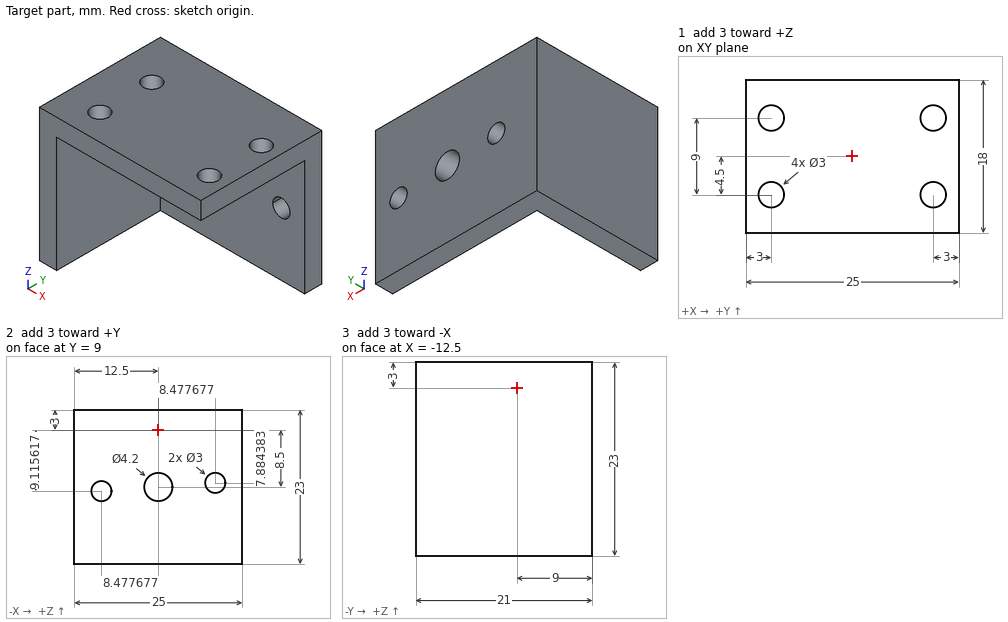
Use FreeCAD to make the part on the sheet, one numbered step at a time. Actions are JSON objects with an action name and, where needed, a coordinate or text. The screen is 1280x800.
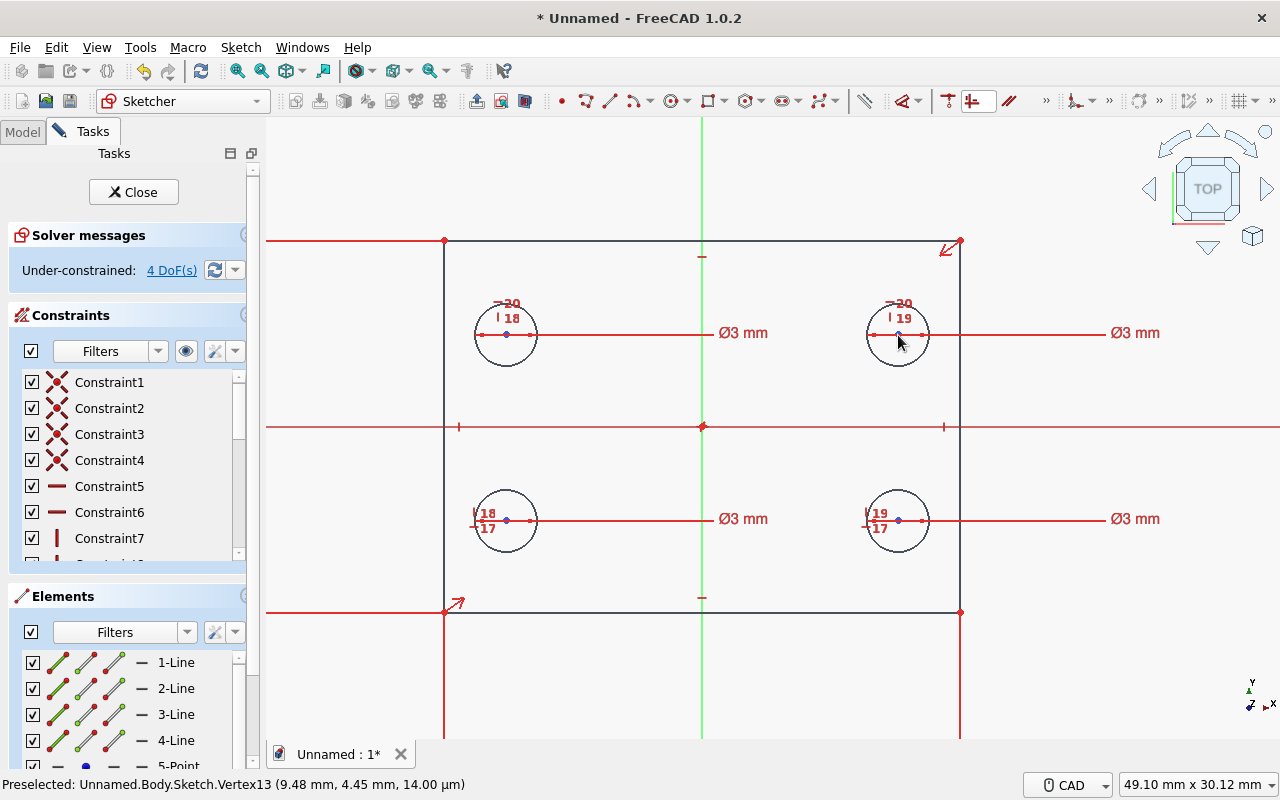
{"action": "key", "text": "d"}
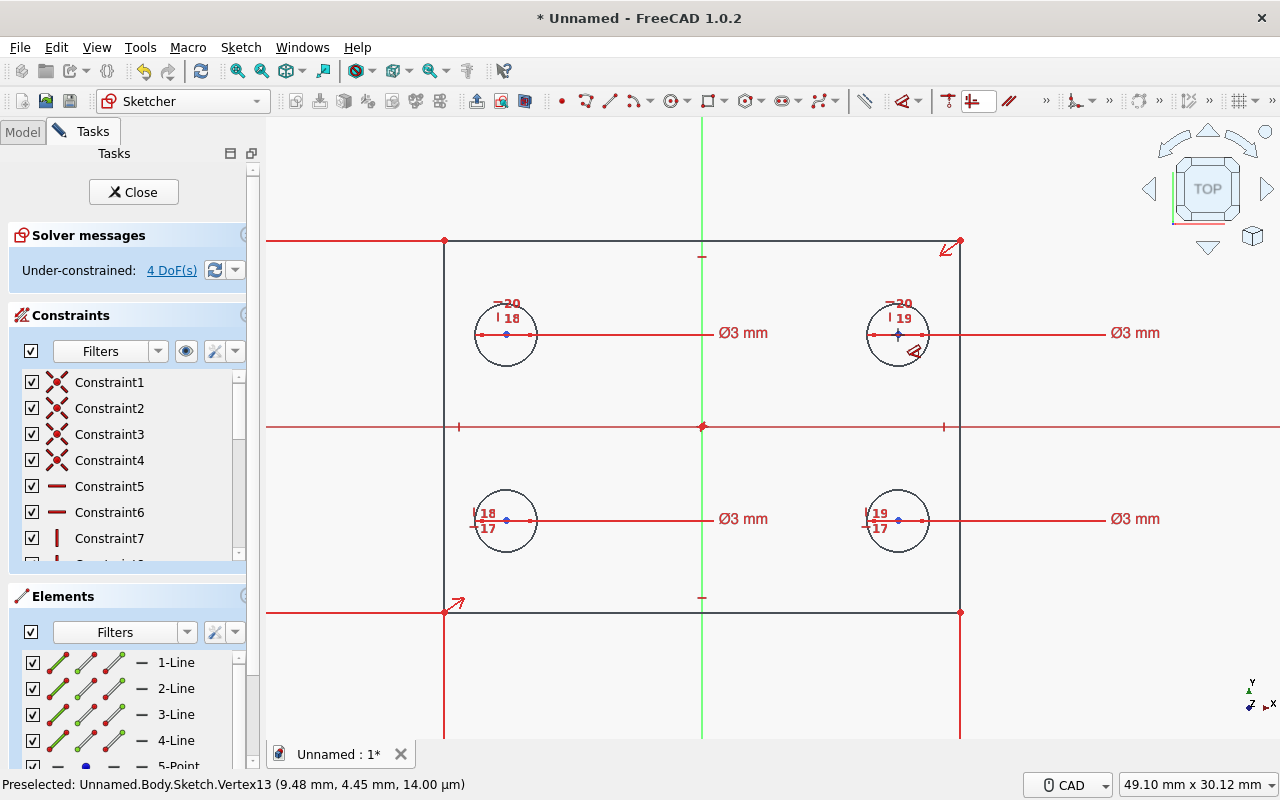
{"action": "left_click", "coordinate": [444, 613]}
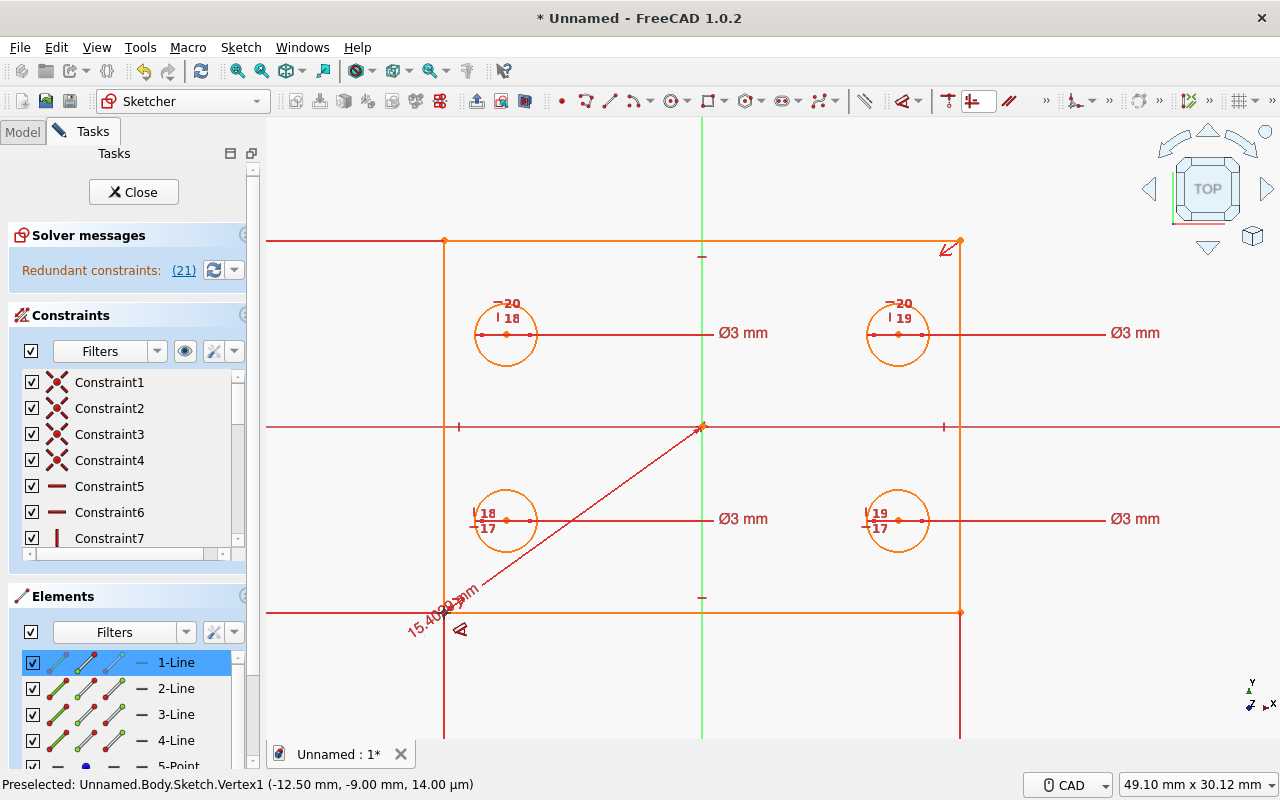
{"action": "left_click", "coordinate": [506, 521]}
{"action": "left_click", "coordinate": [475, 647]}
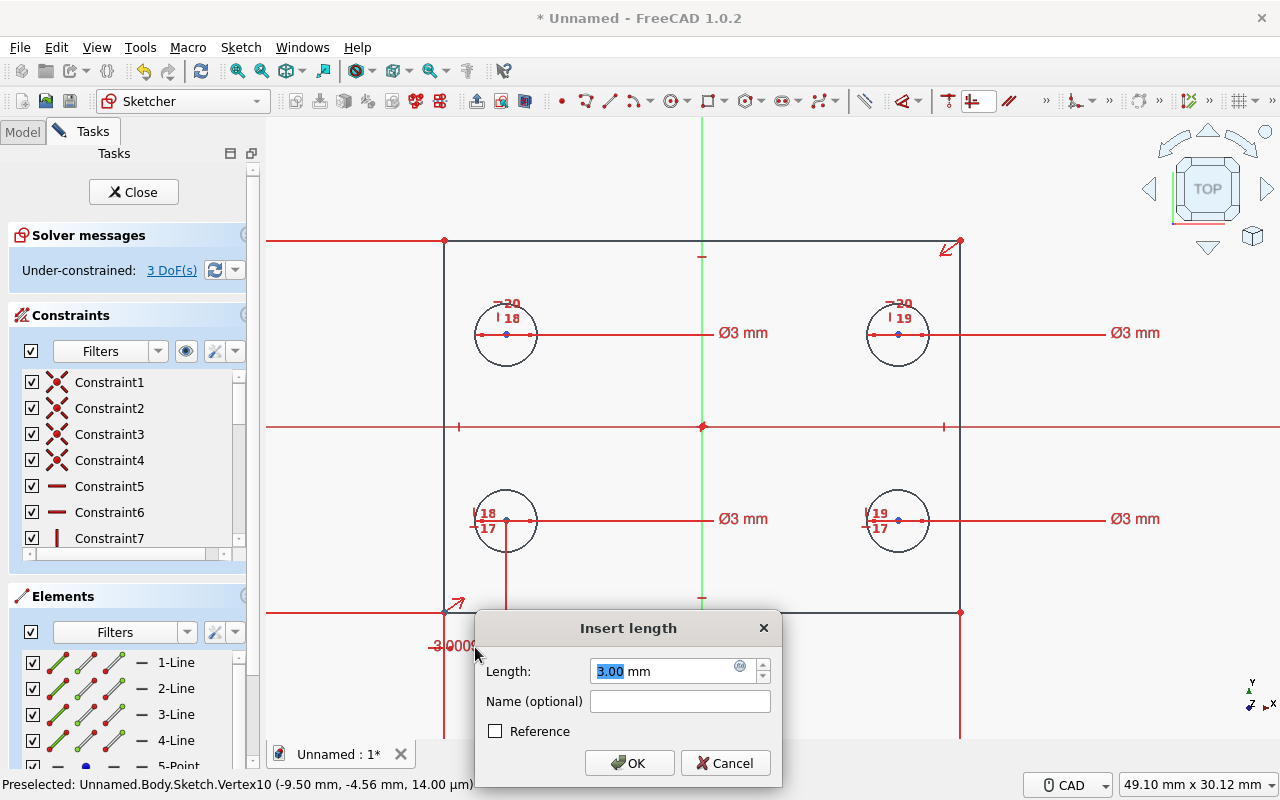
{"action": "type", "text": "3"}
{"action": "key", "text": "Return"}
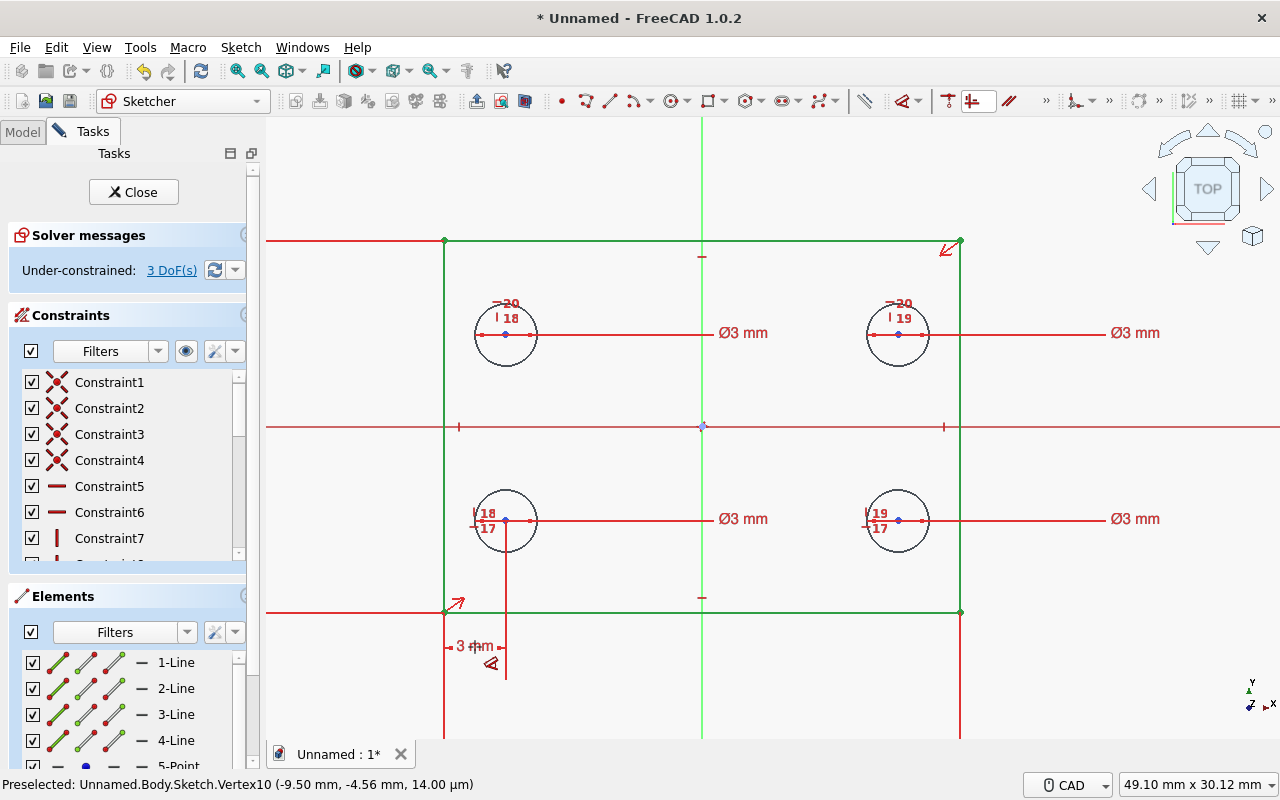
{"action": "left_click", "coordinate": [960, 613]}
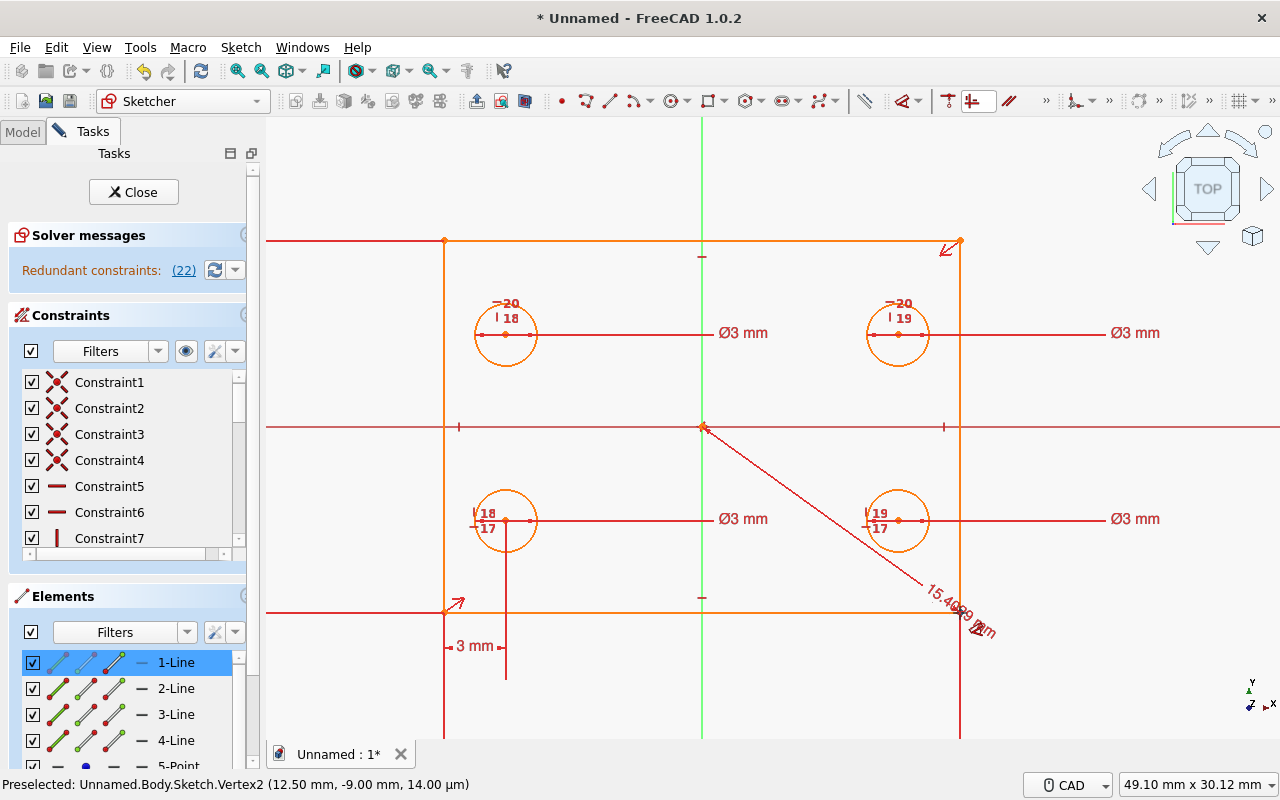
{"action": "left_click", "coordinate": [898, 521]}
{"action": "left_click", "coordinate": [929, 647]}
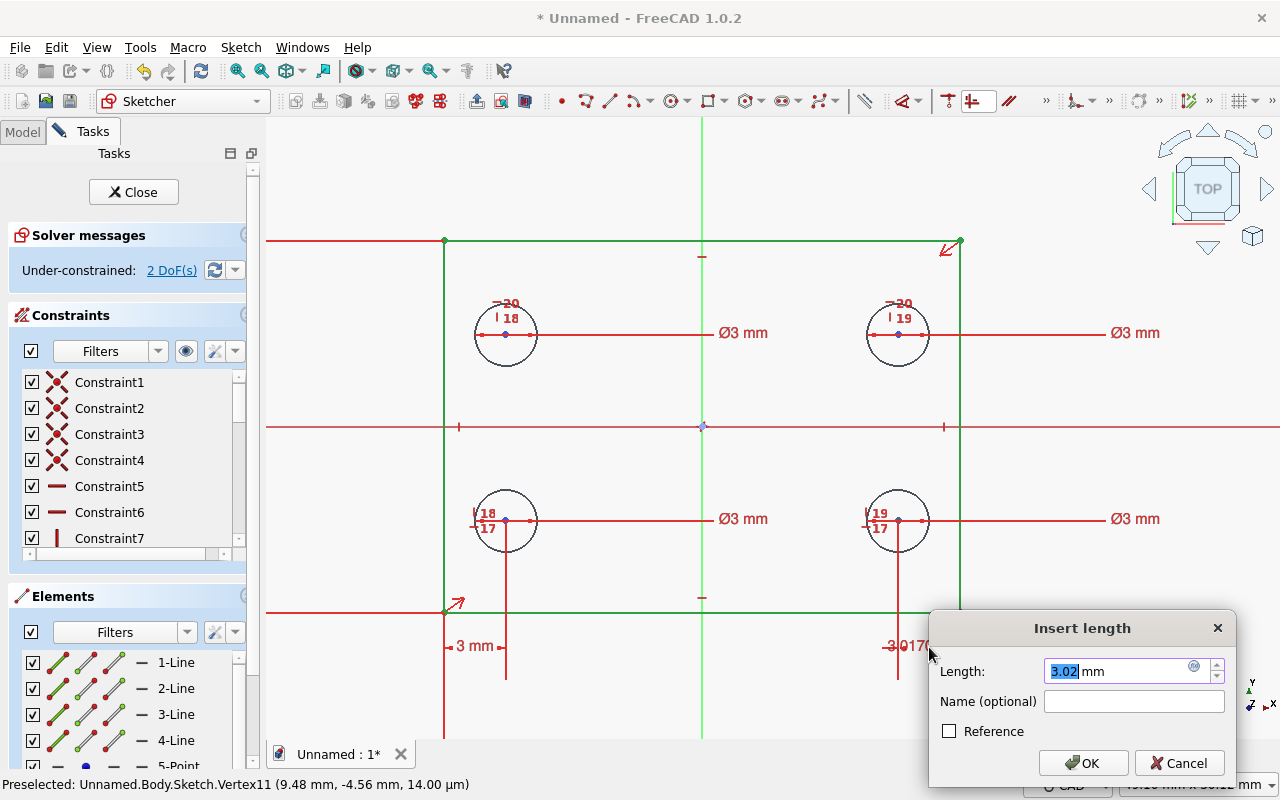
{"action": "type", "text": "3"}
{"action": "key", "text": "Return"}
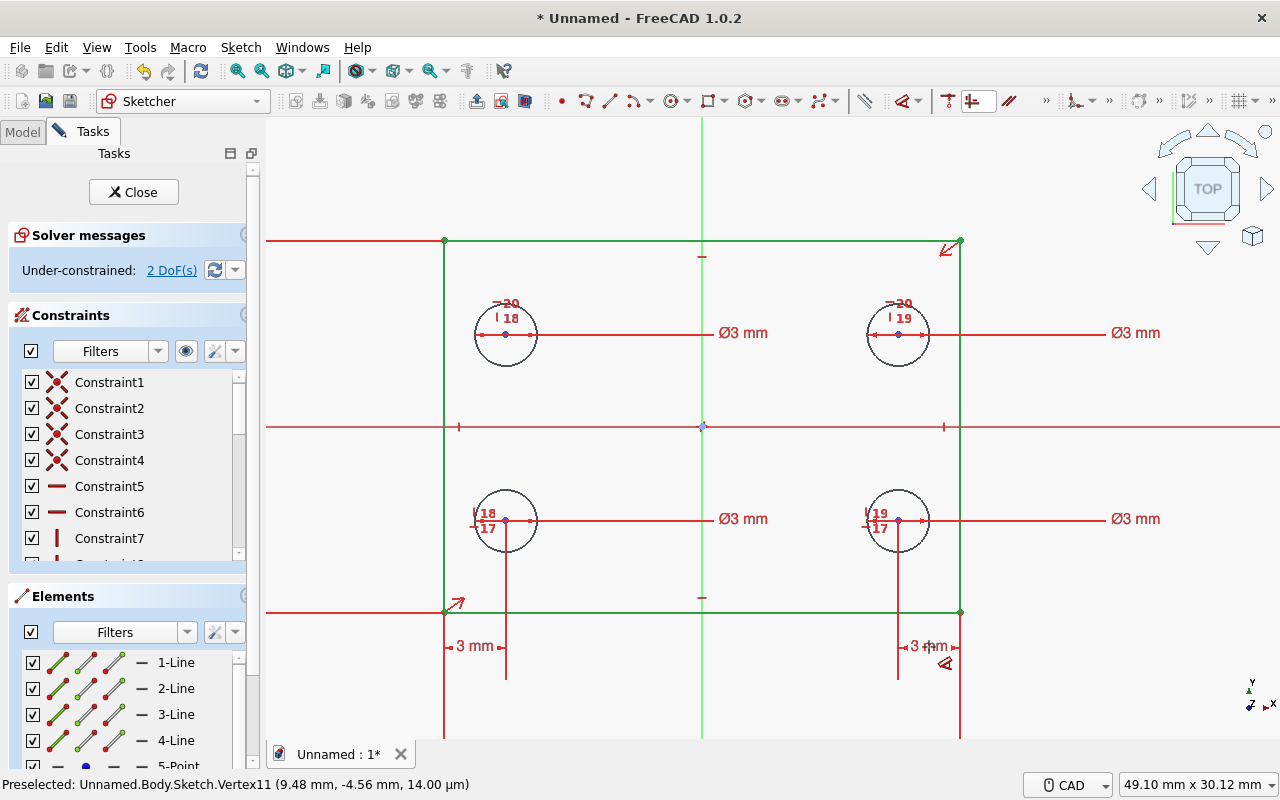
{"action": "left_click", "coordinate": [506, 521]}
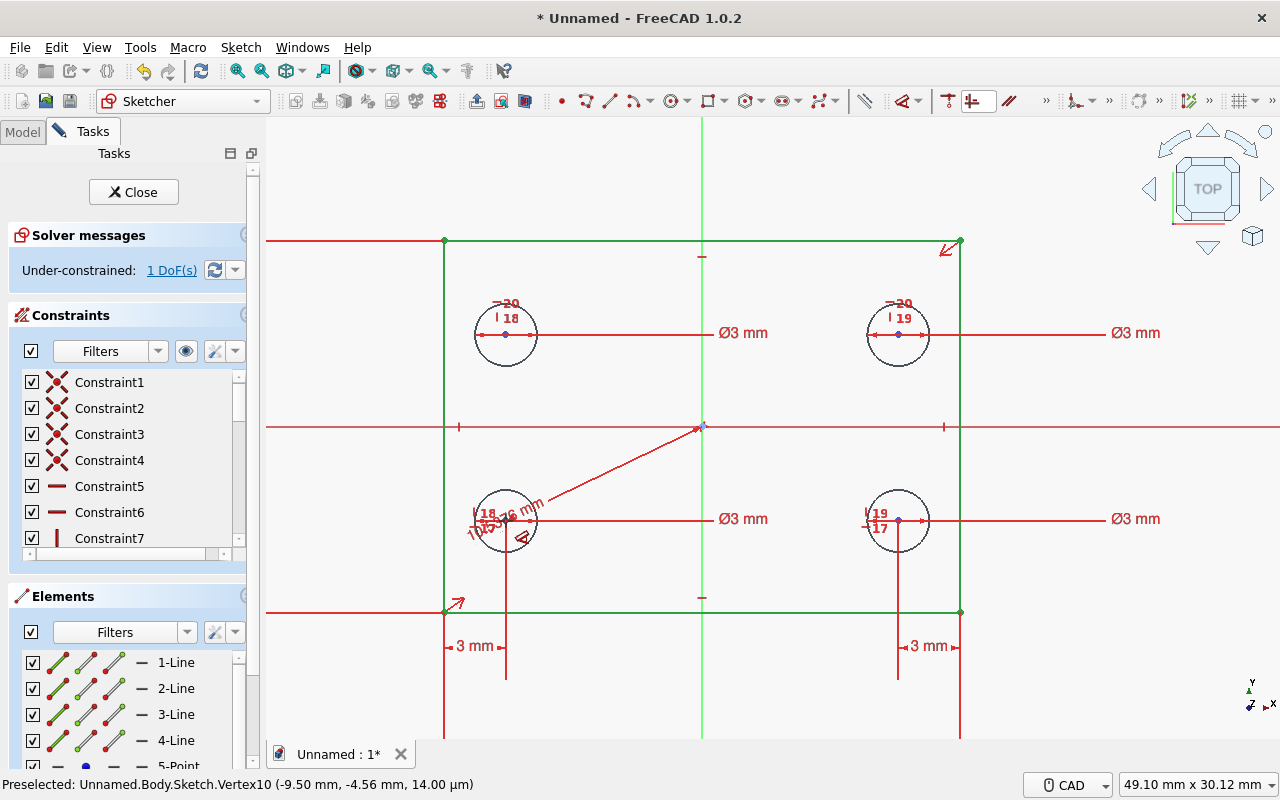
{"action": "left_click", "coordinate": [506, 335]}
{"action": "left_click", "coordinate": [472, 385]}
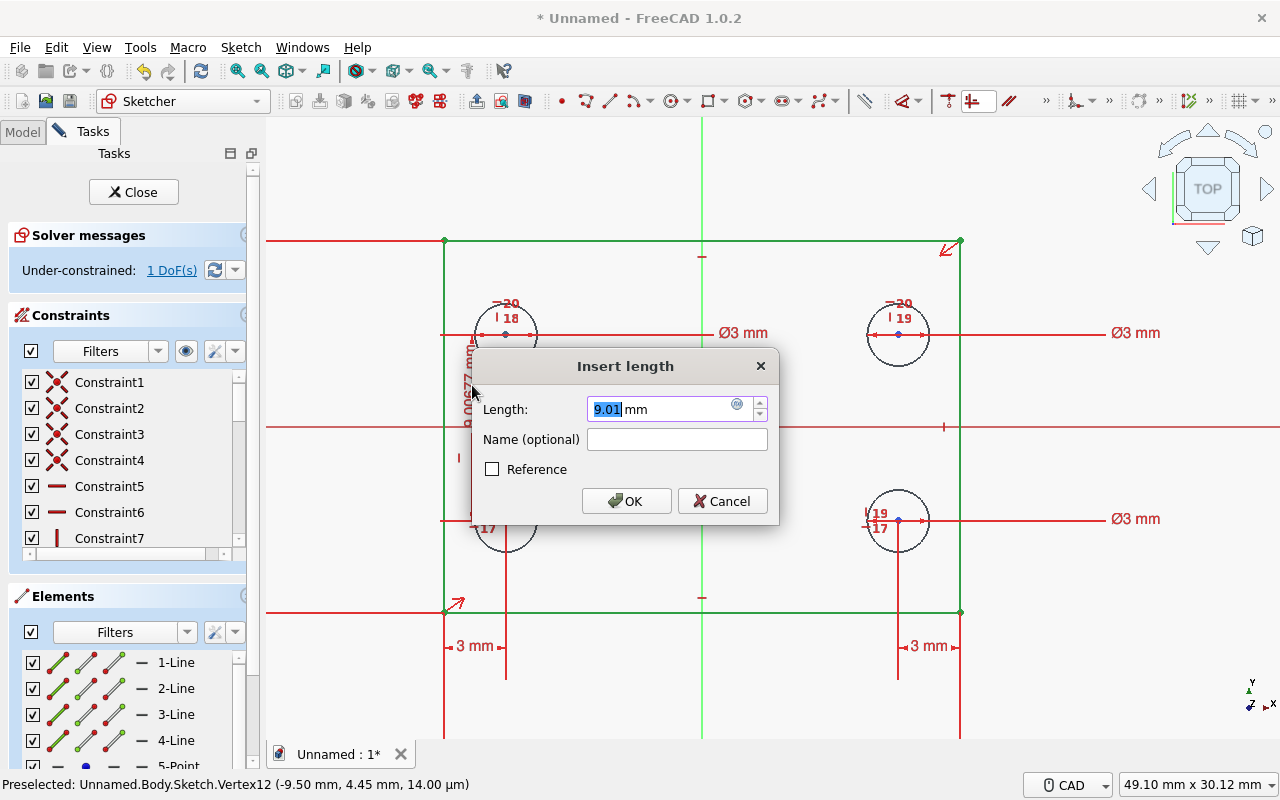
{"action": "type", "text": "9"}
{"action": "key", "text": "Return"}